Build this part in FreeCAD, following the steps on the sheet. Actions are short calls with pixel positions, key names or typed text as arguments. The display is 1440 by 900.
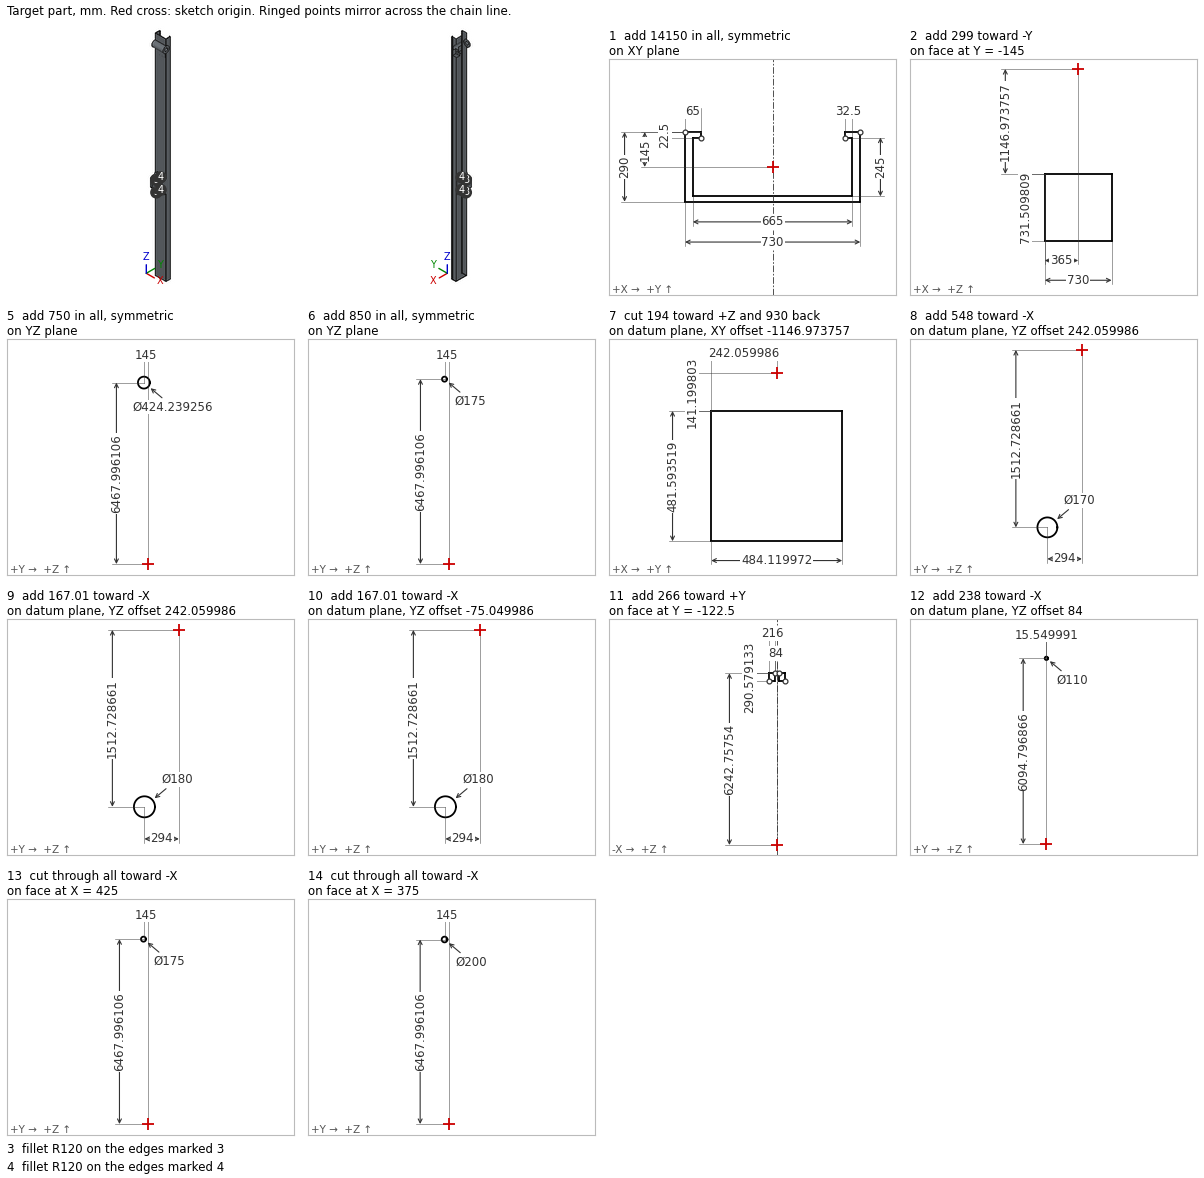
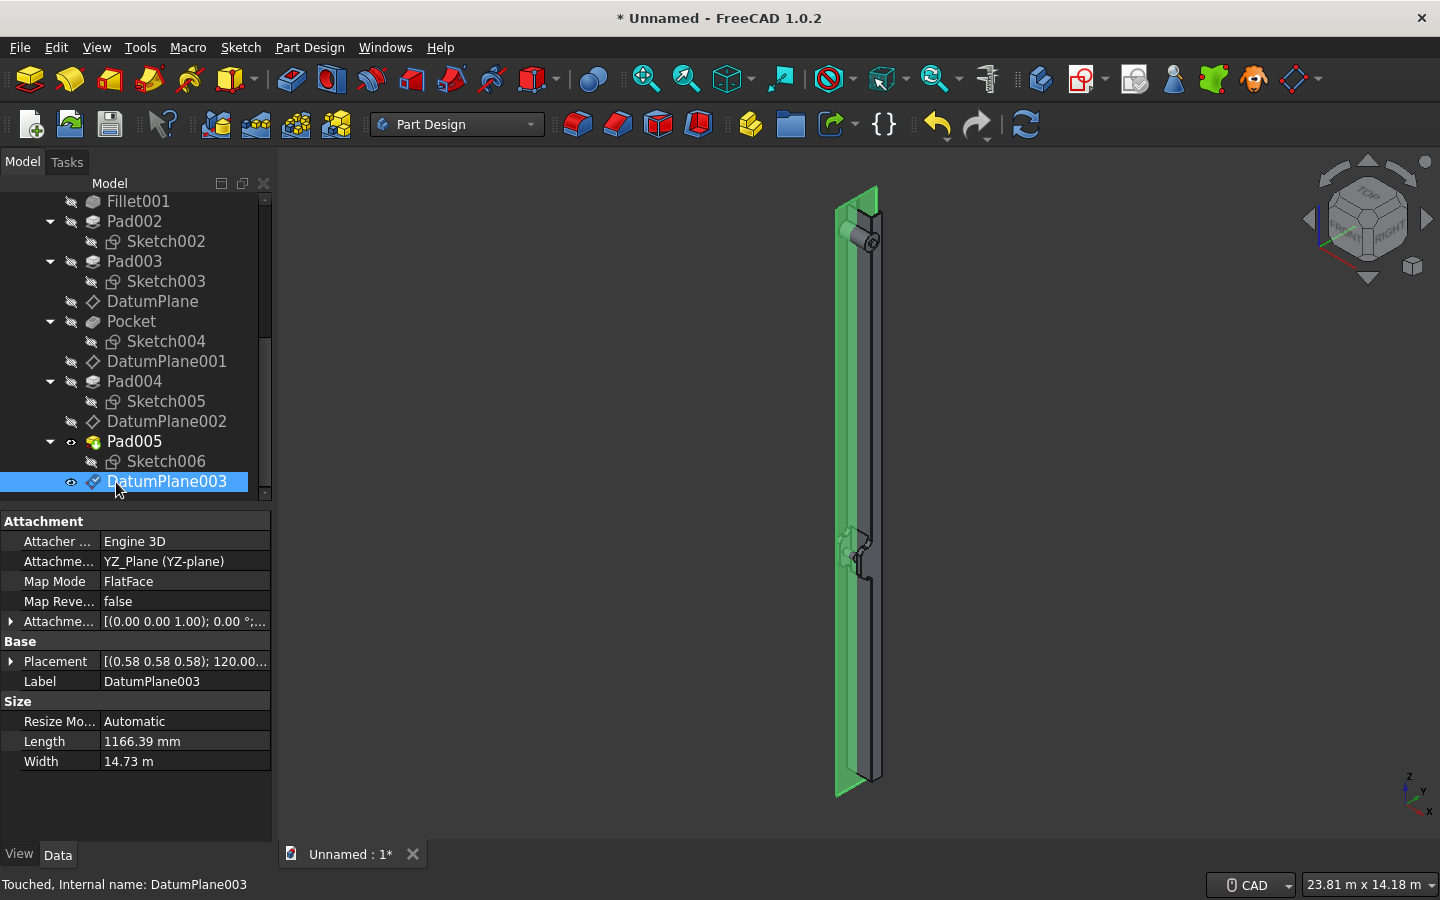
click(1082, 80)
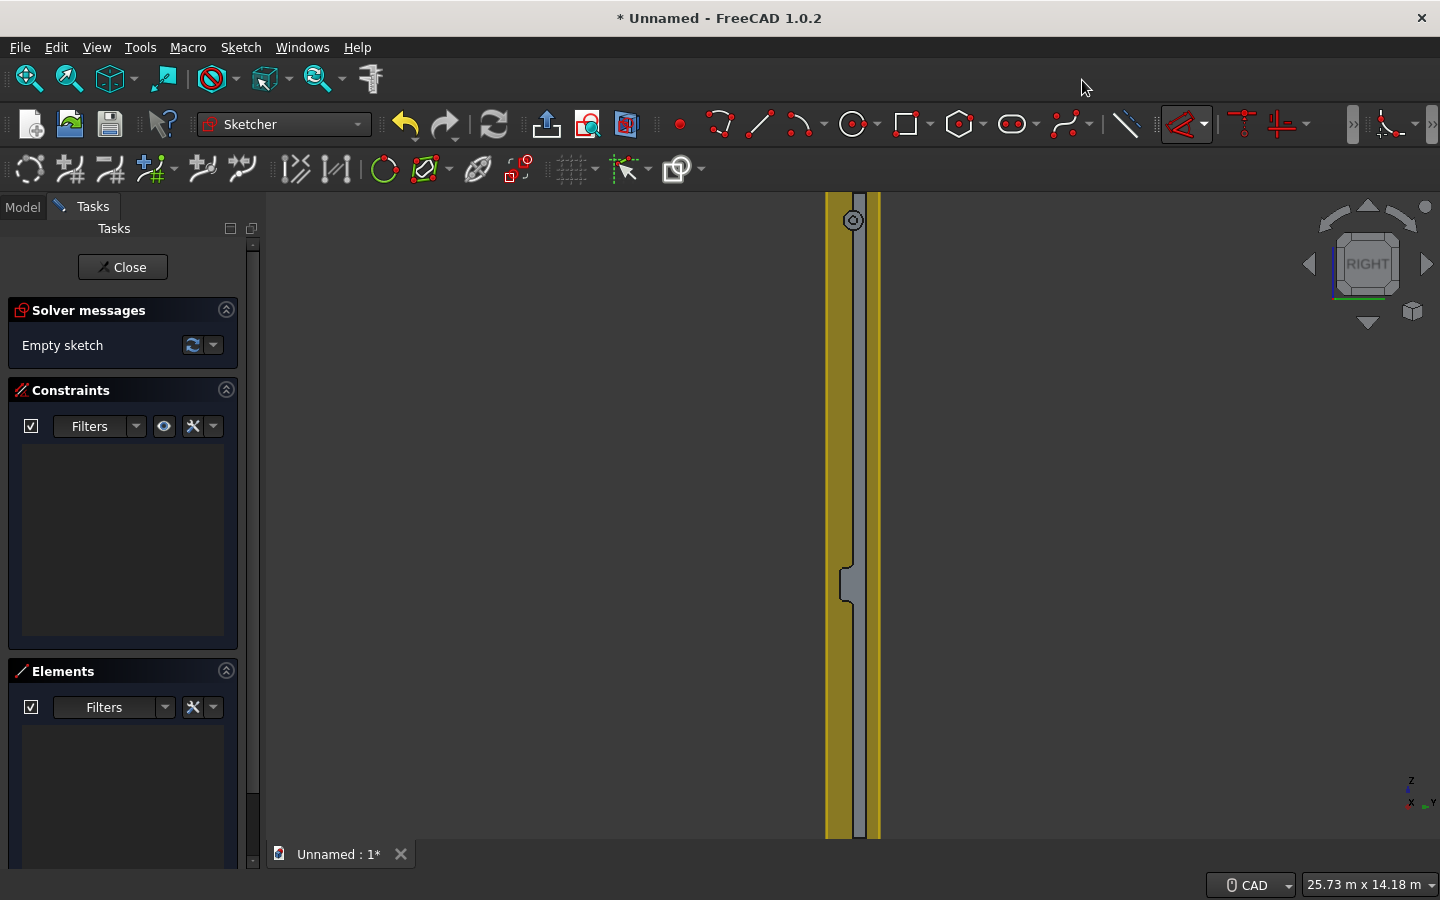
click(628, 124)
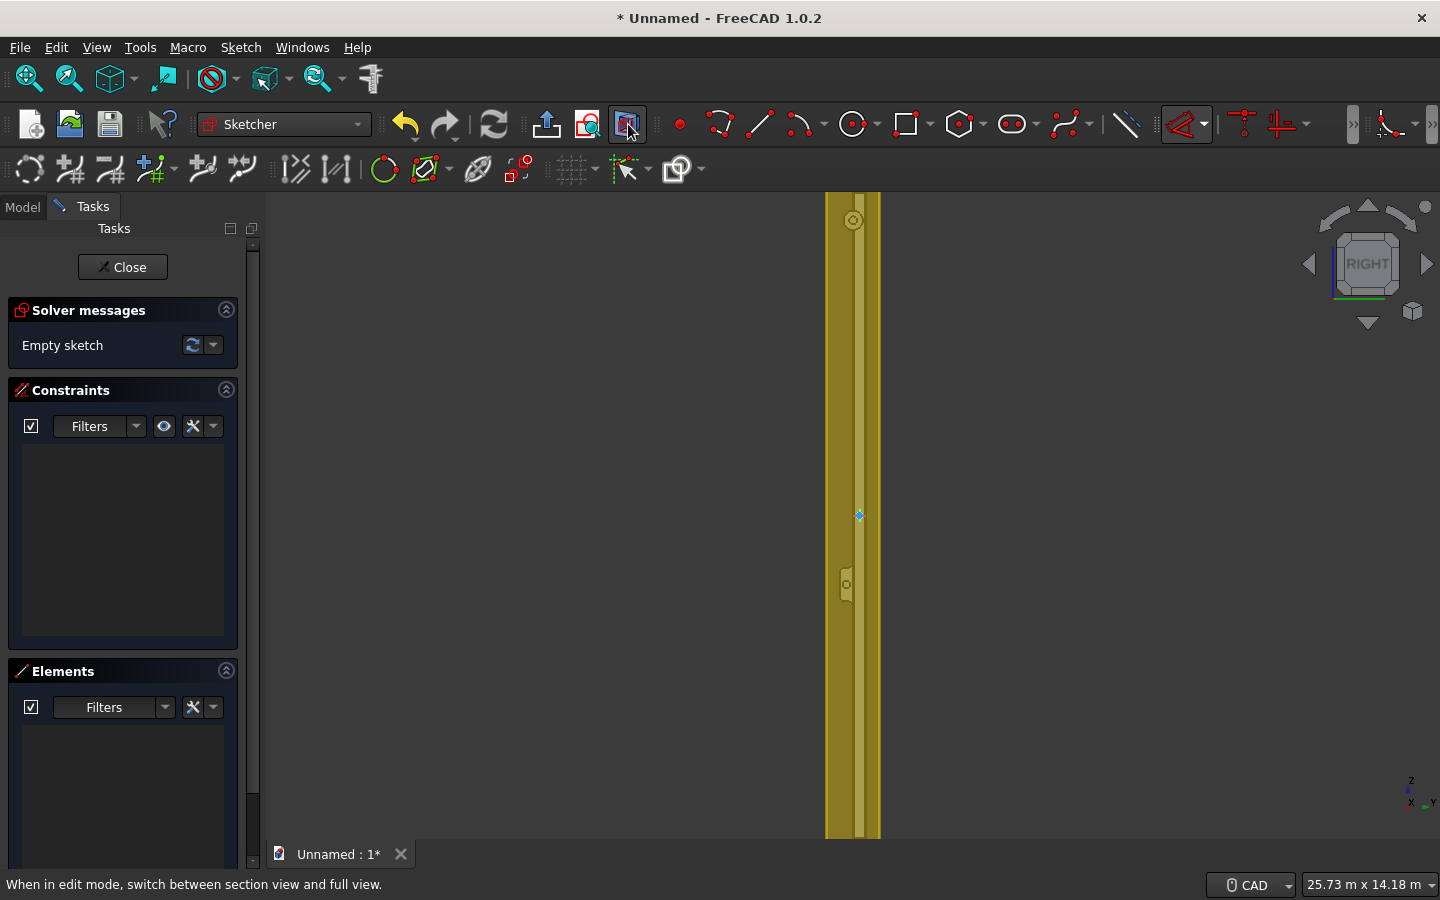
scroll(850, 588, up, 15)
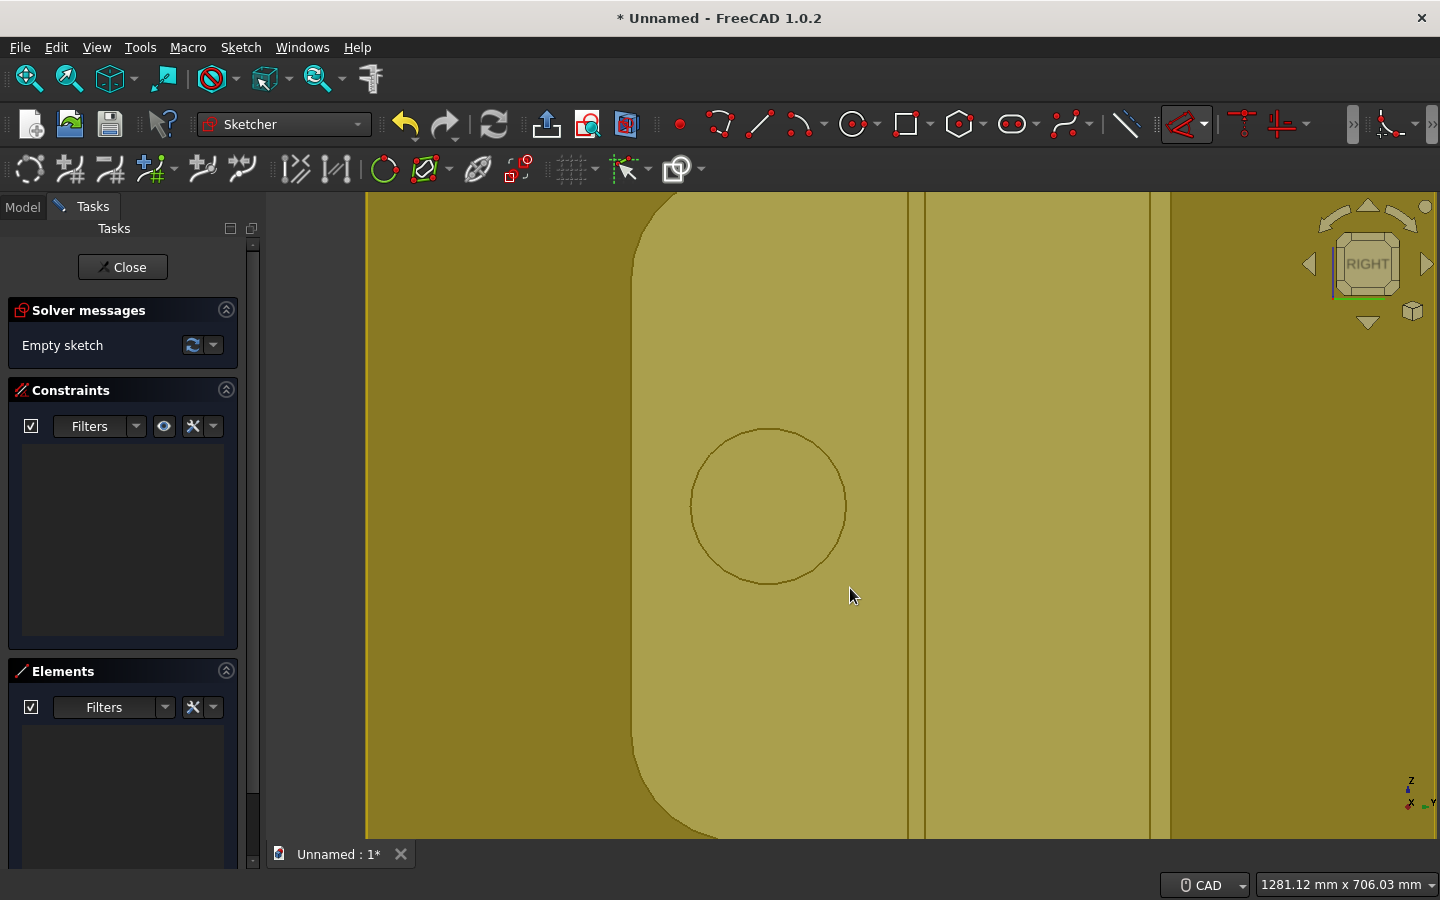
scroll(759, 501, up, 5)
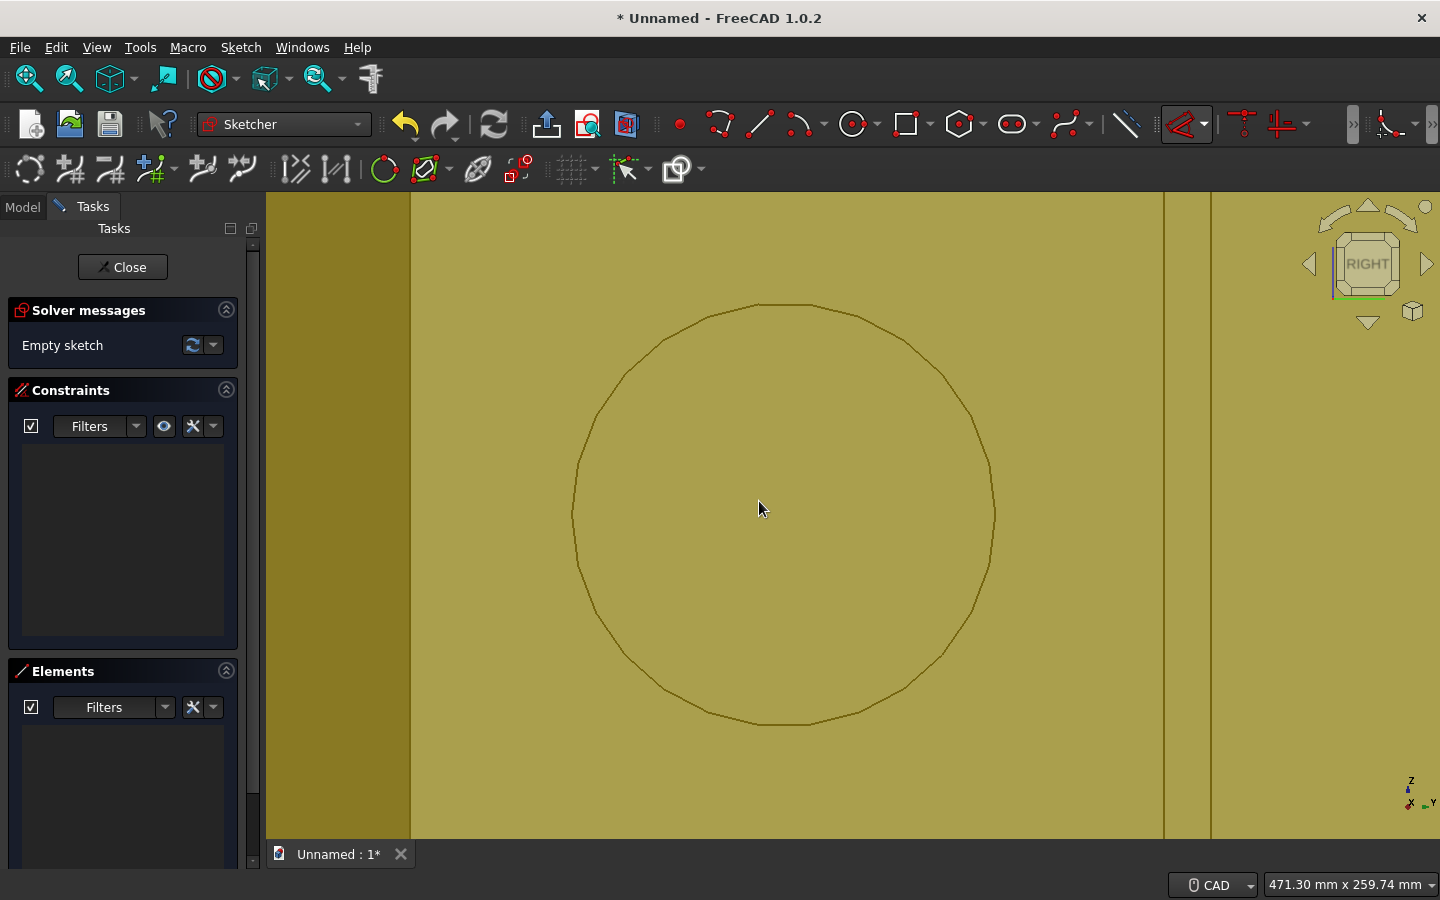
click(854, 124)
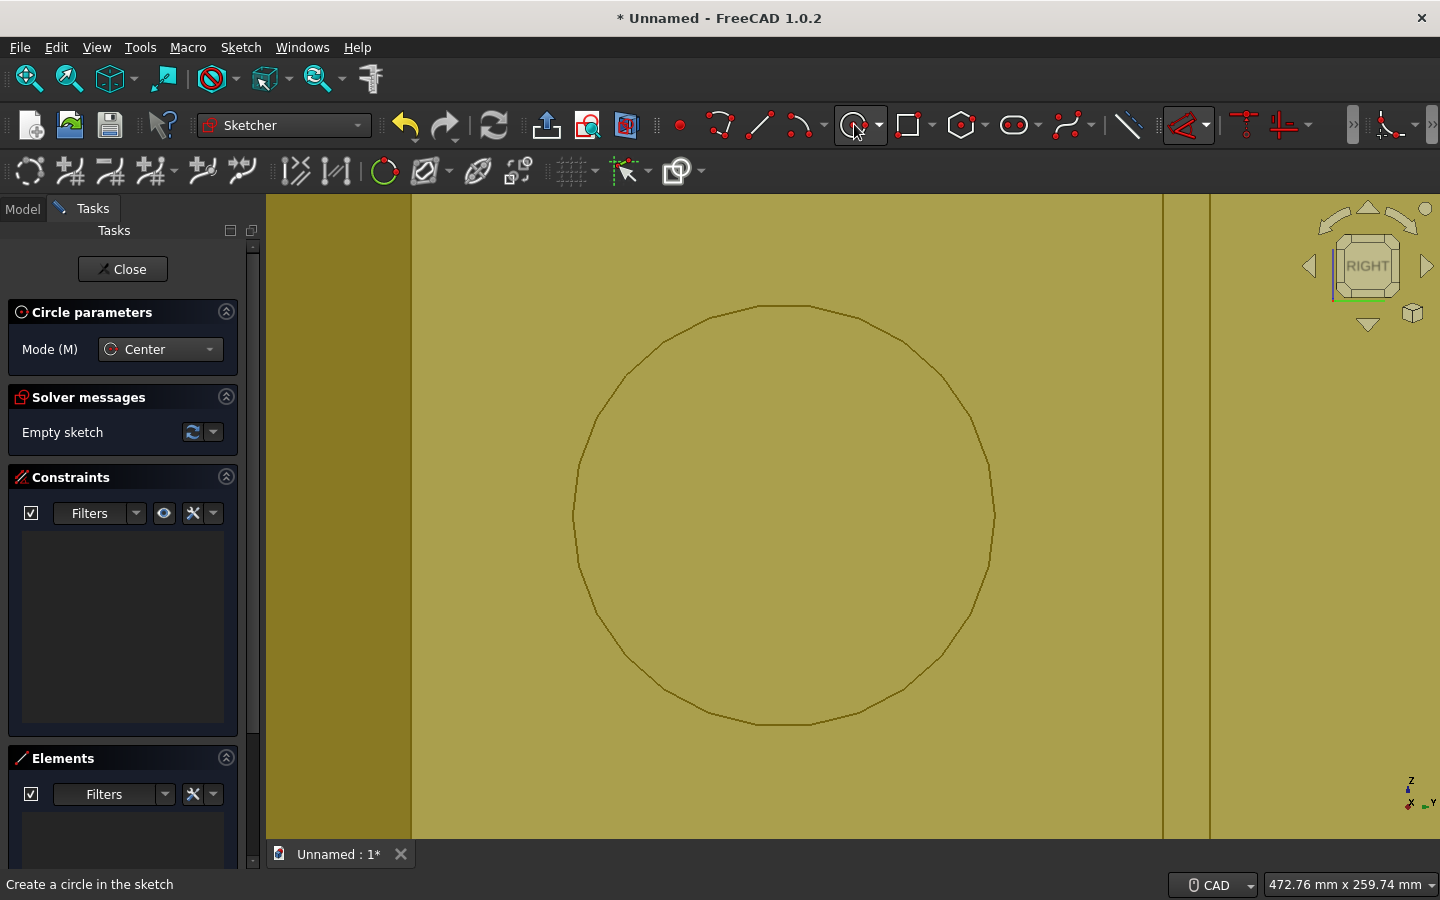
click(784, 516)
click(942, 358)
key(Escape)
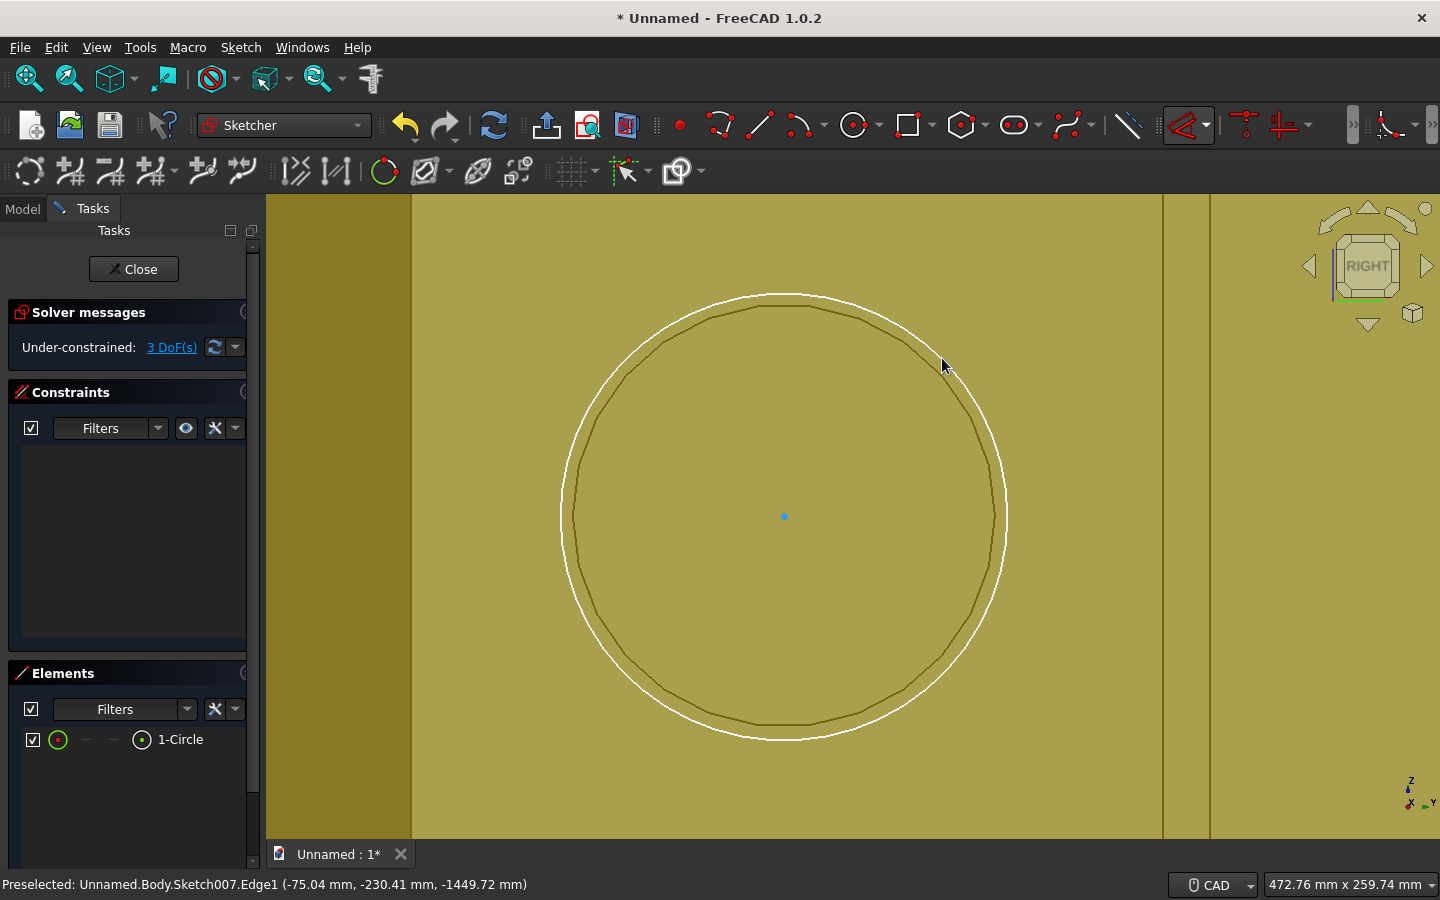
click(942, 359)